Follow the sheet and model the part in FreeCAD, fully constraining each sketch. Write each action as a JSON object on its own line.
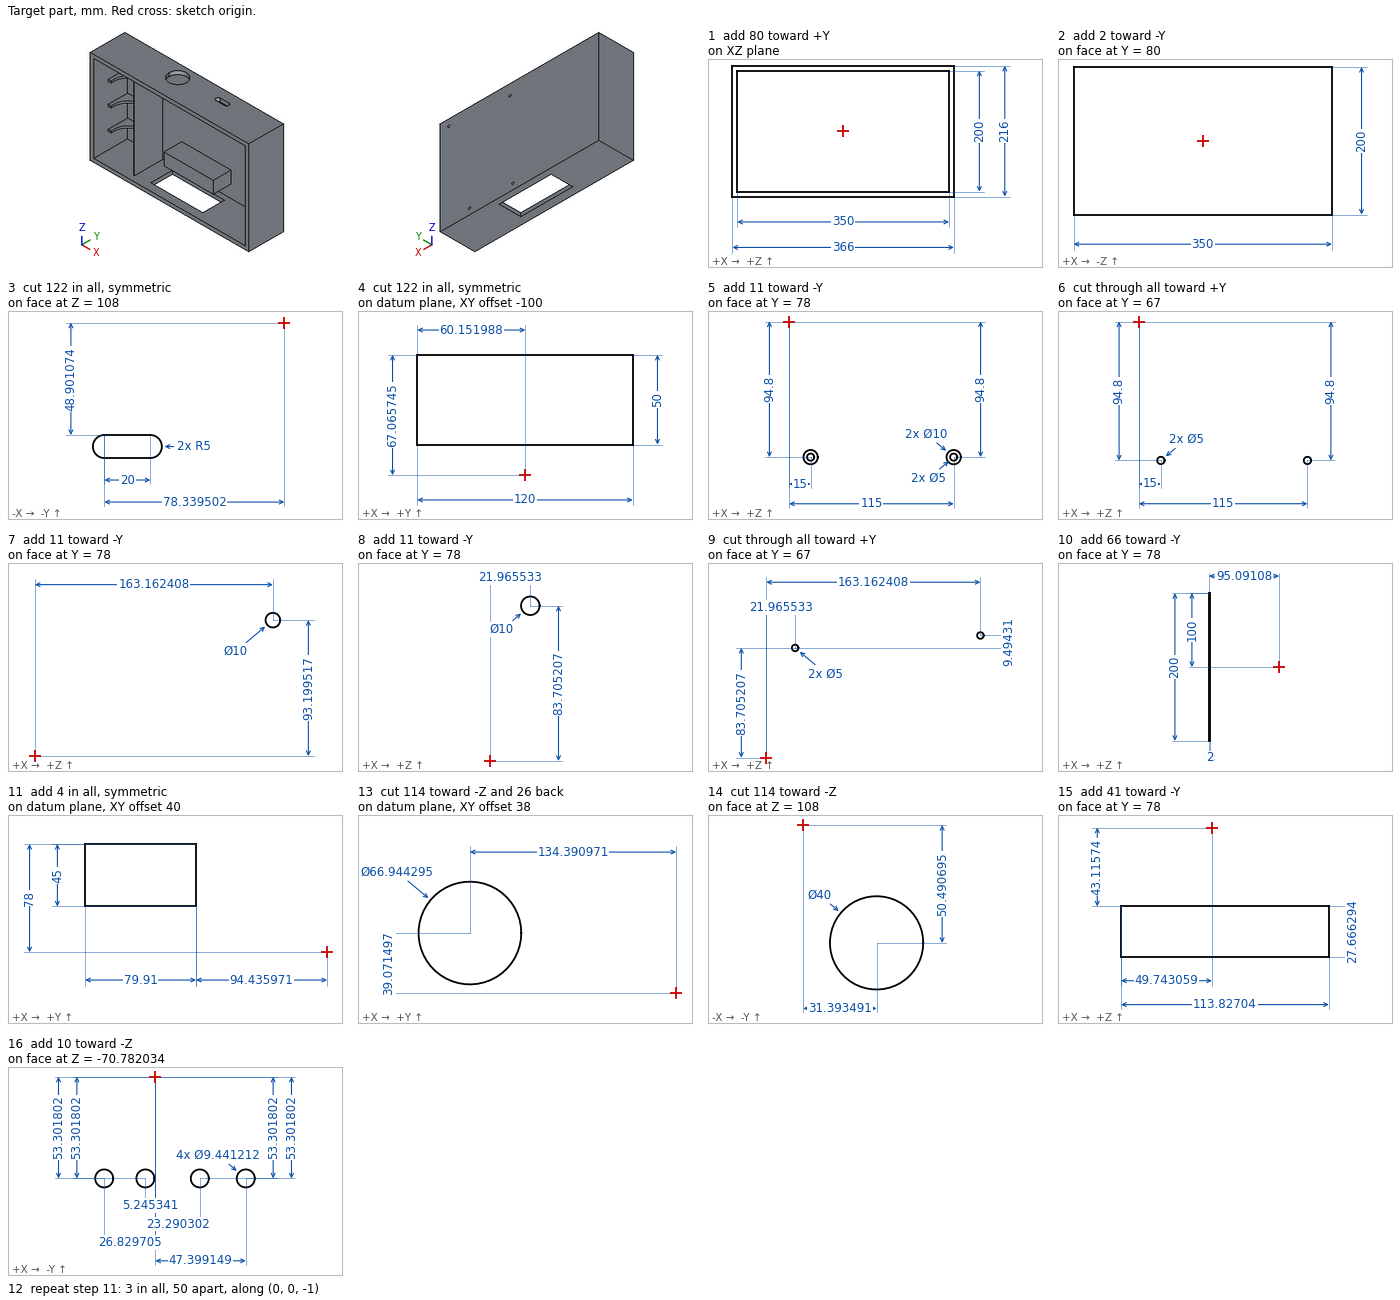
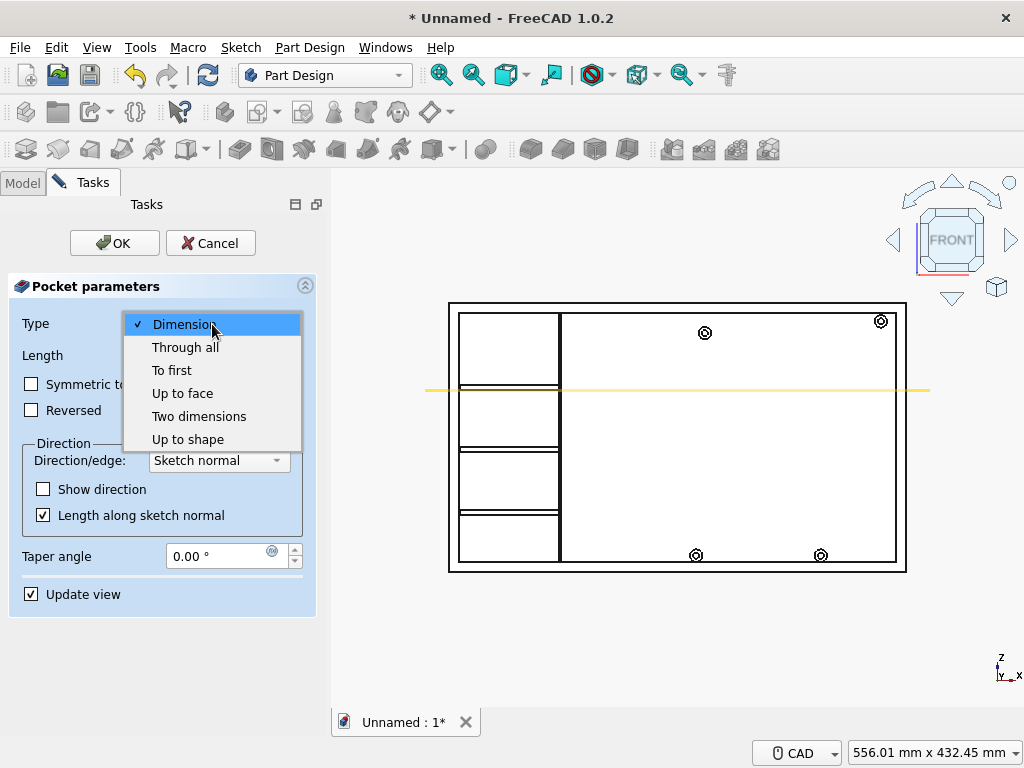
{"action": "left_click", "coordinate": [212, 416]}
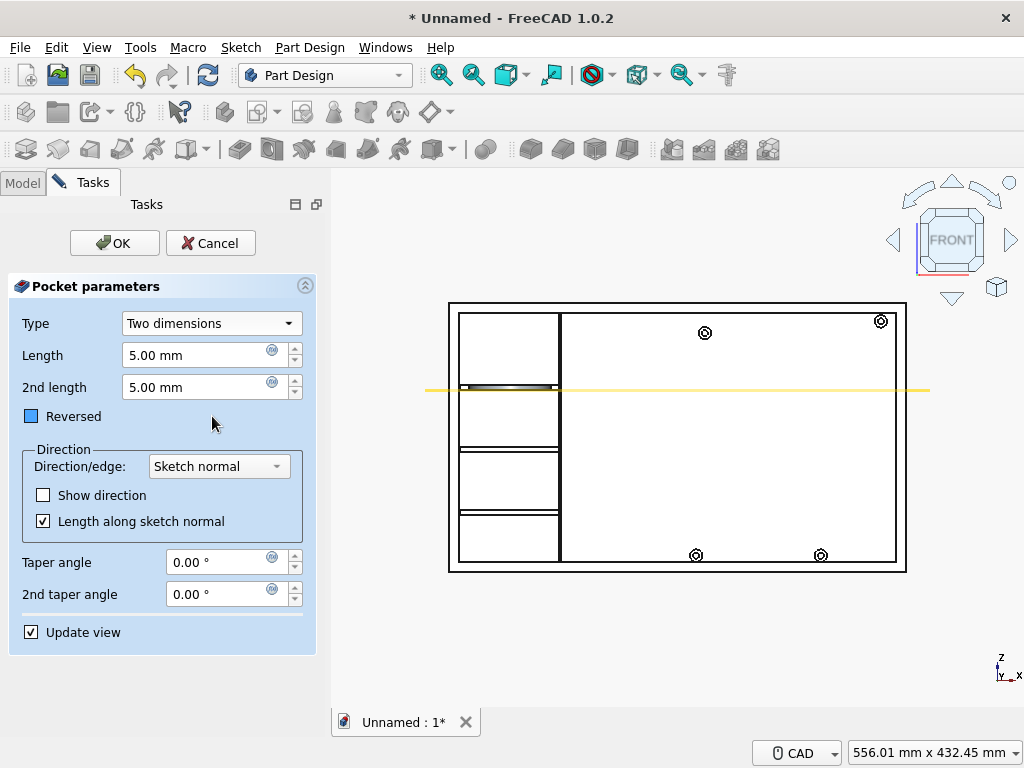
{"action": "triple_click", "coordinate": [204, 355]}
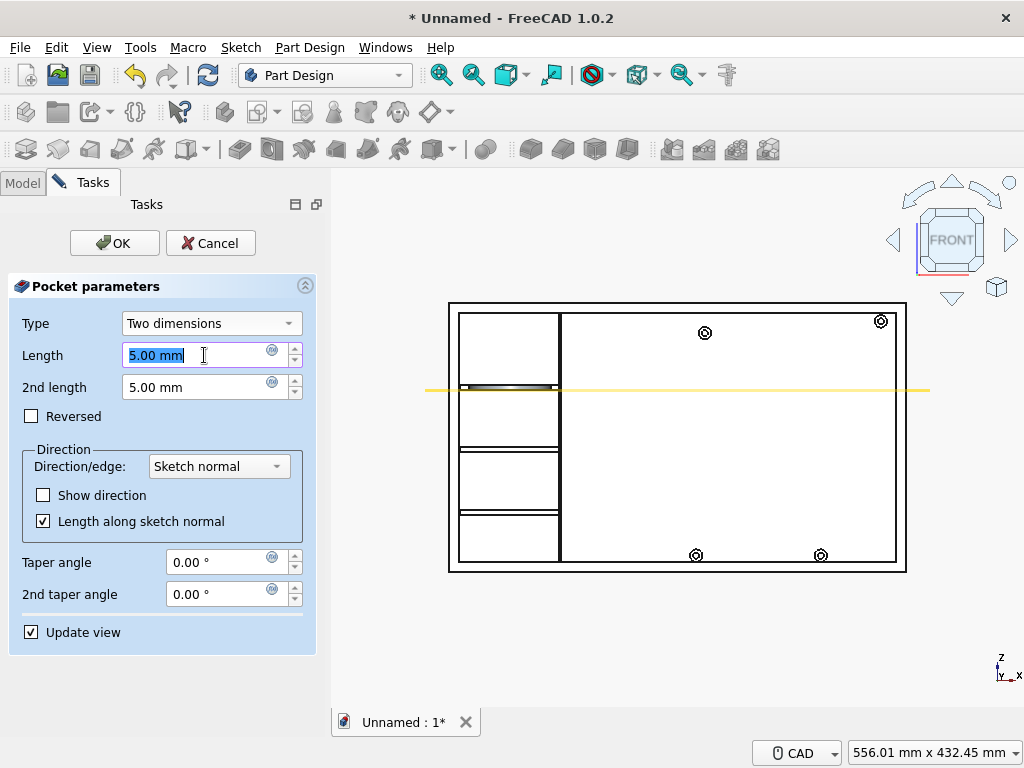
{"action": "type", "text": "114"}
{"action": "key", "text": "Tab"}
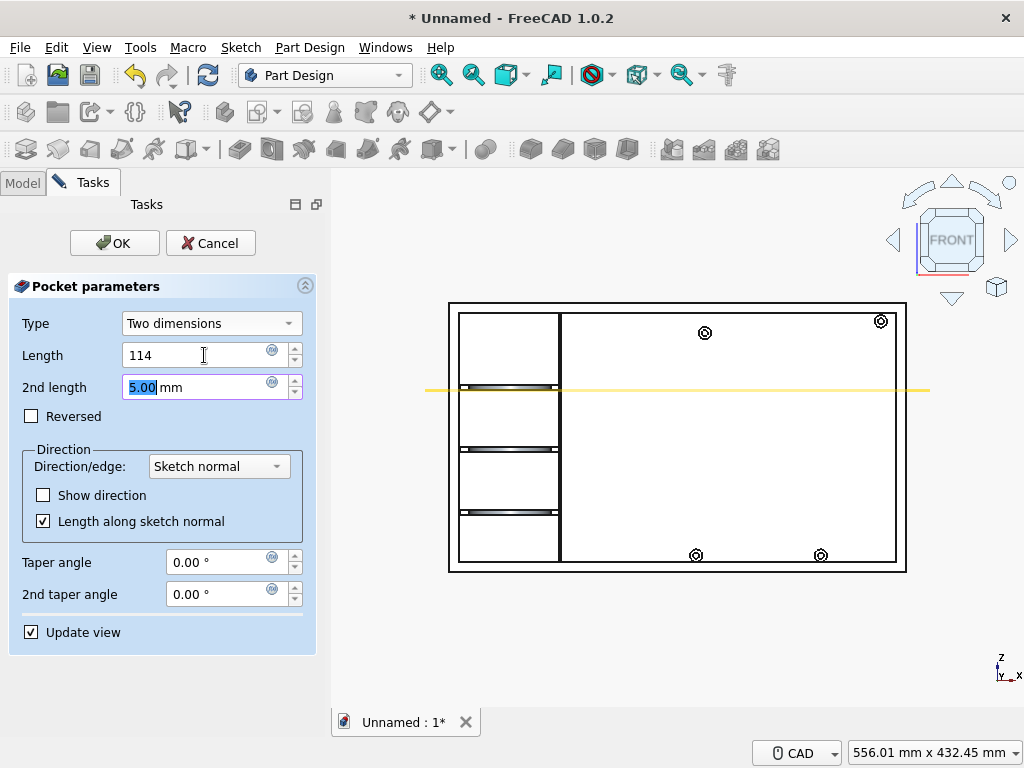
{"action": "type", "text": "26"}
{"action": "key", "text": "Tab"}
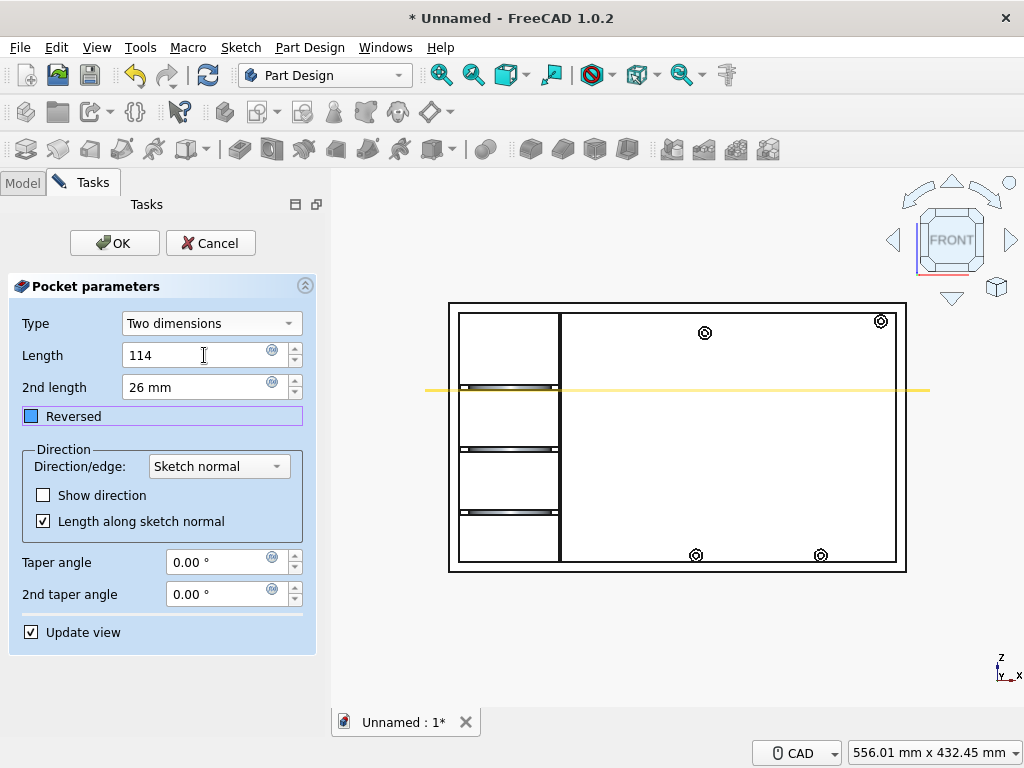
{"action": "left_click", "coordinate": [115, 243]}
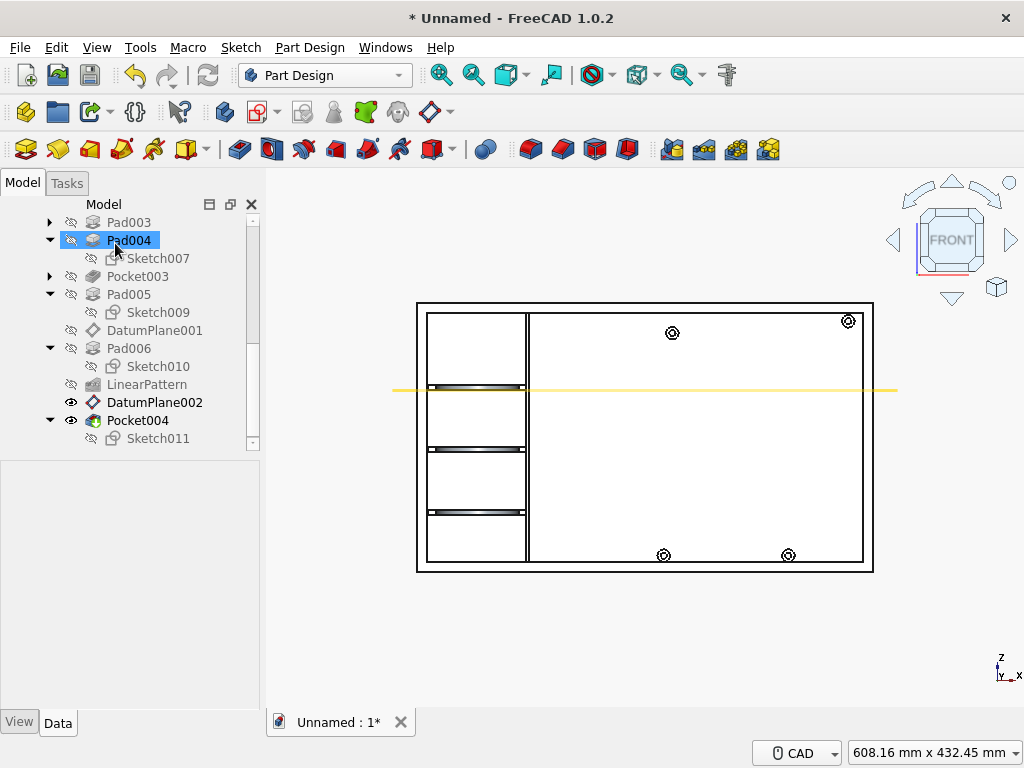
{"action": "left_click", "coordinate": [116, 402]}
{"action": "key", "text": "space"}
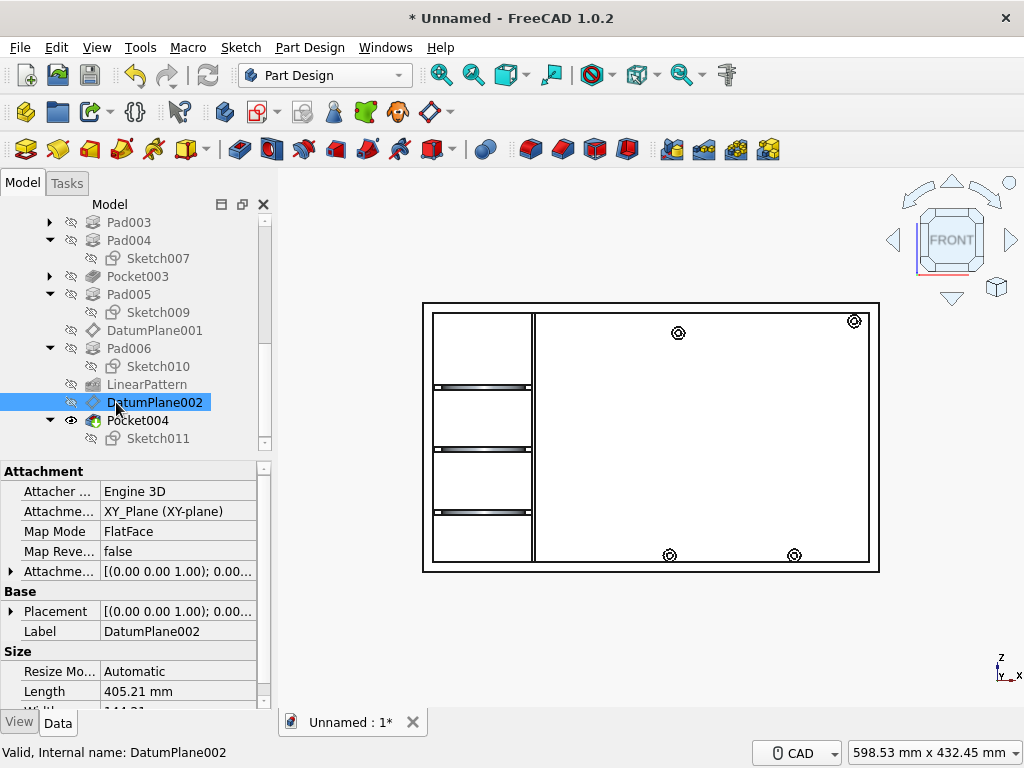
{"action": "key", "text": "0"}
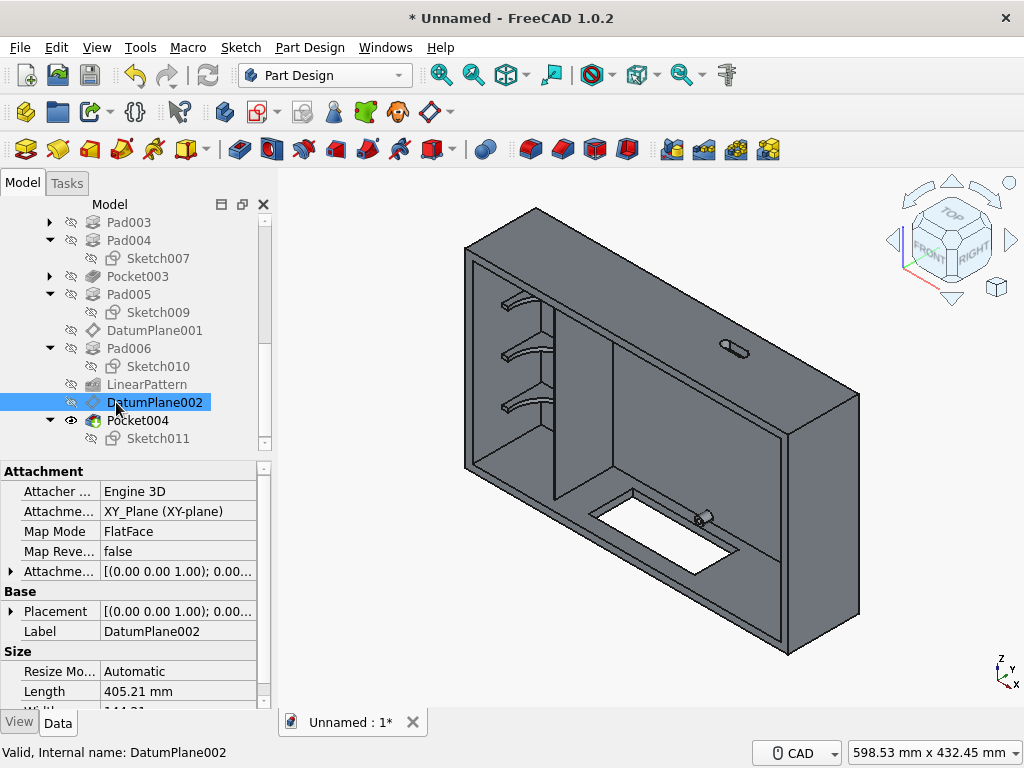
{"action": "left_click", "coordinate": [662, 320]}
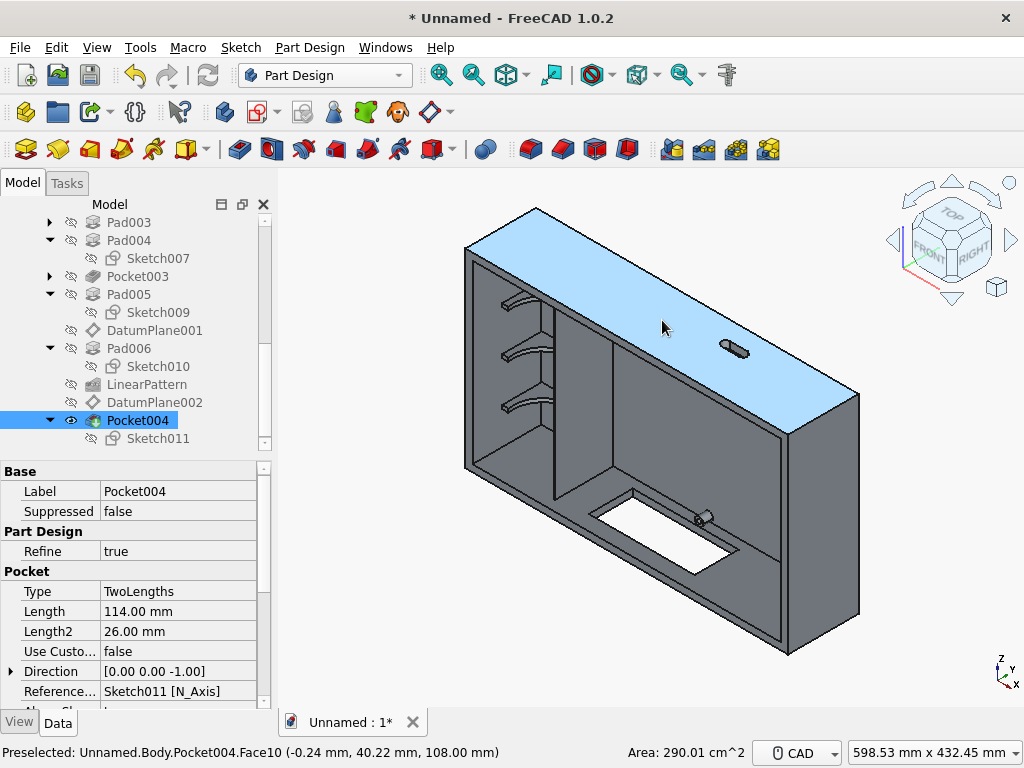
{"action": "left_click", "coordinate": [258, 112]}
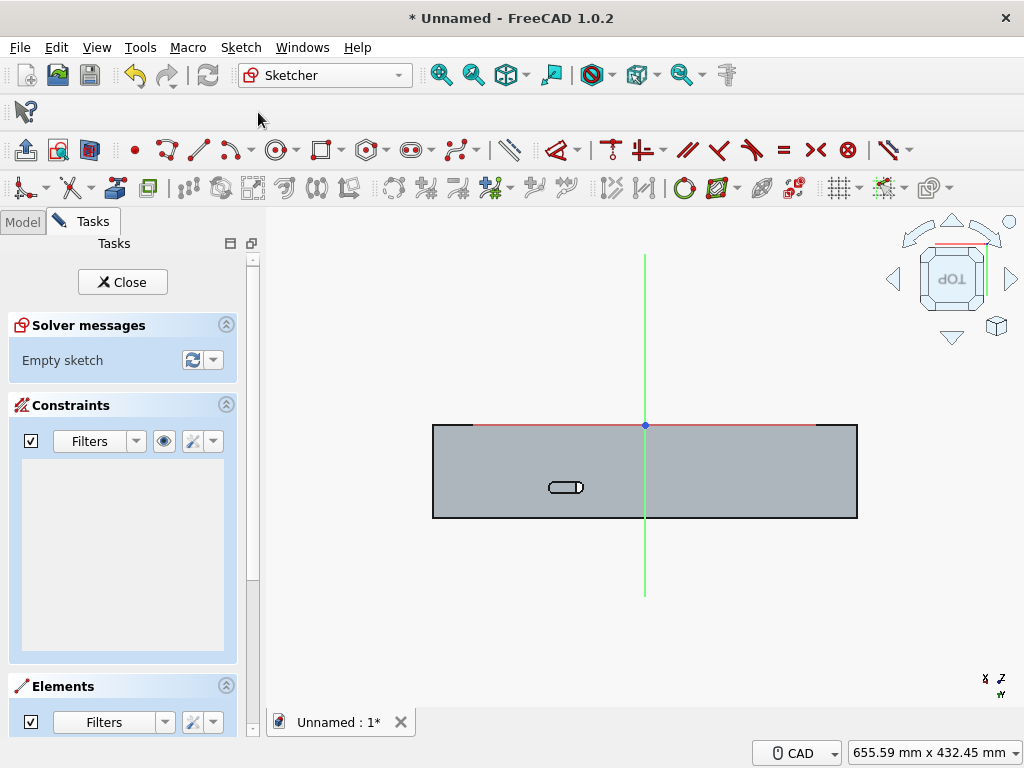
{"action": "scroll", "coordinate": [707, 469], "scroll_direction": "up", "scroll_amount": 7}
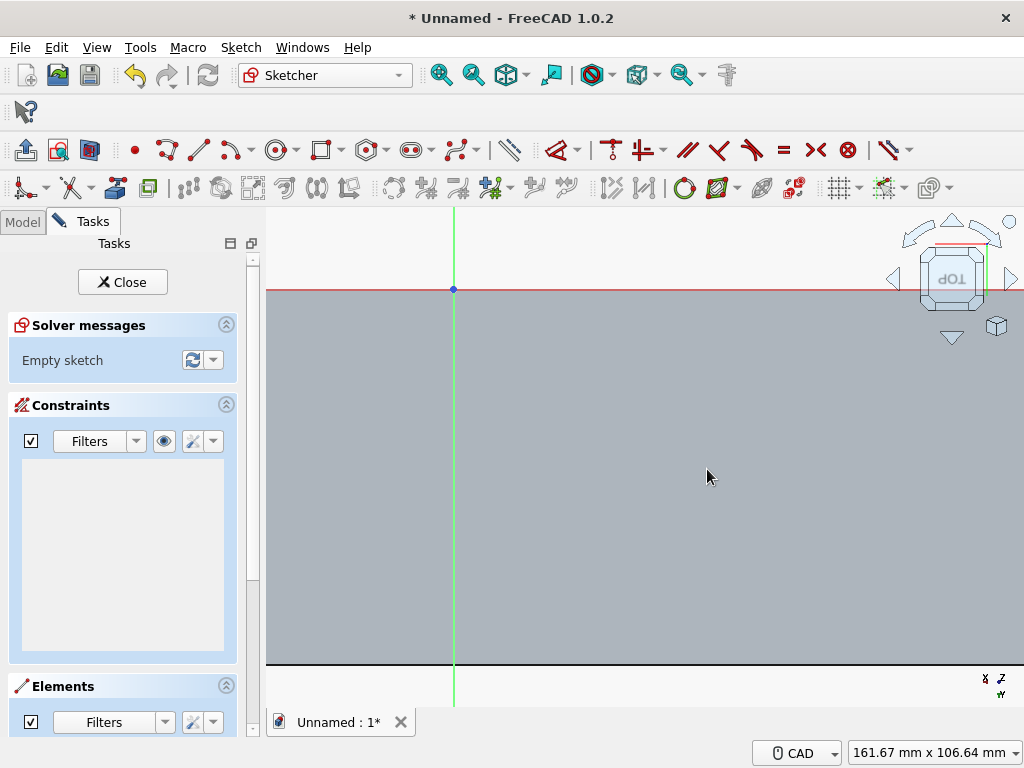
{"action": "key", "text": "g c"}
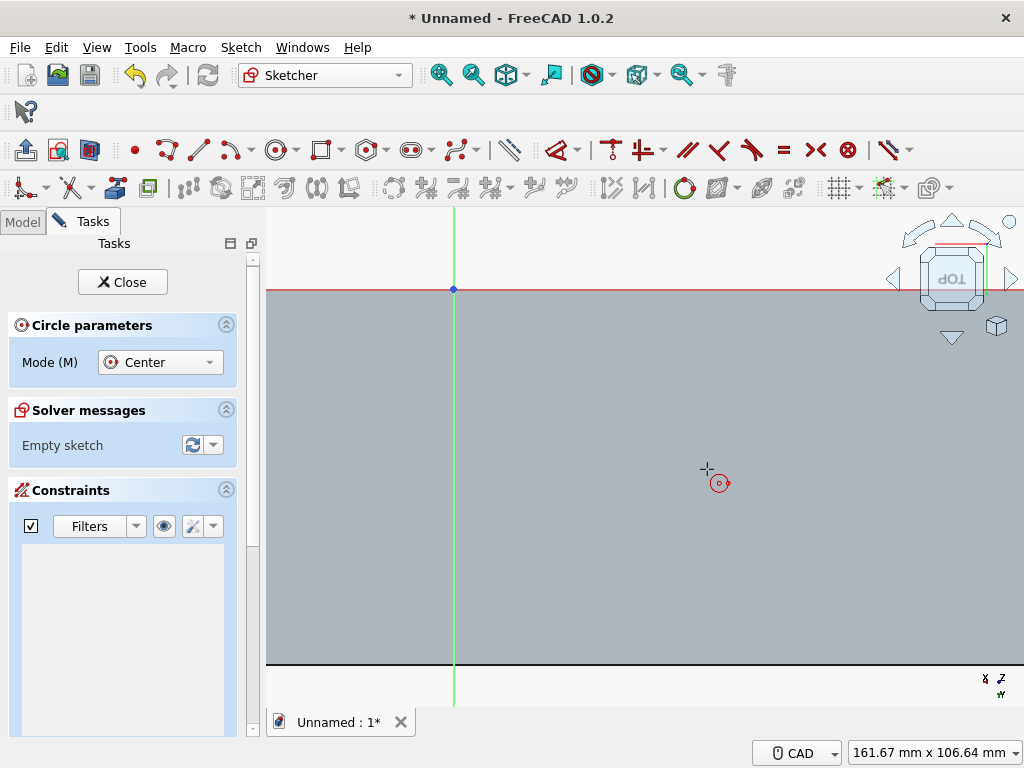
{"action": "left_click", "coordinate": [601, 527]}
{"action": "mouse_move", "coordinate": [667, 460]}